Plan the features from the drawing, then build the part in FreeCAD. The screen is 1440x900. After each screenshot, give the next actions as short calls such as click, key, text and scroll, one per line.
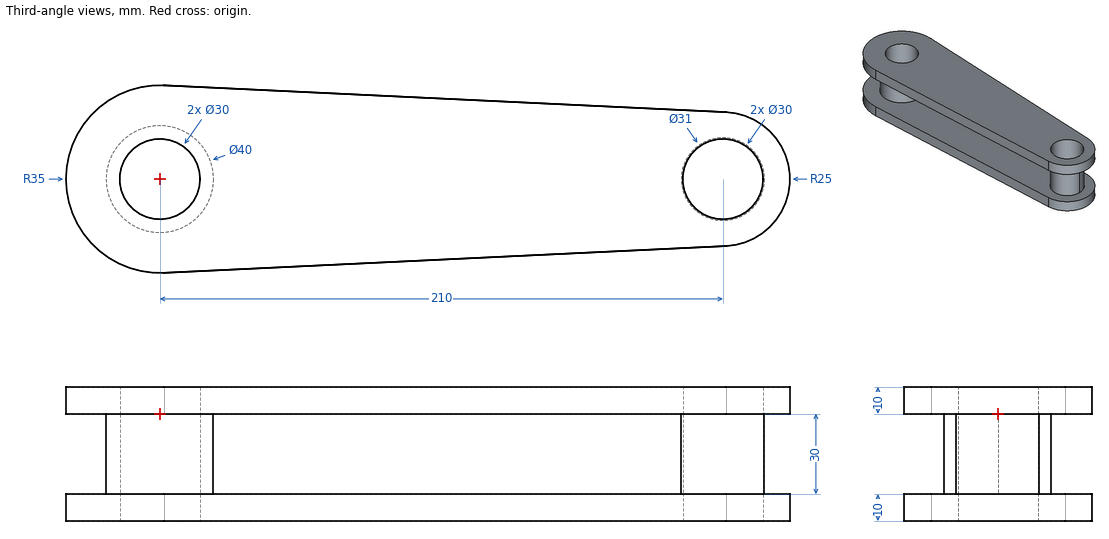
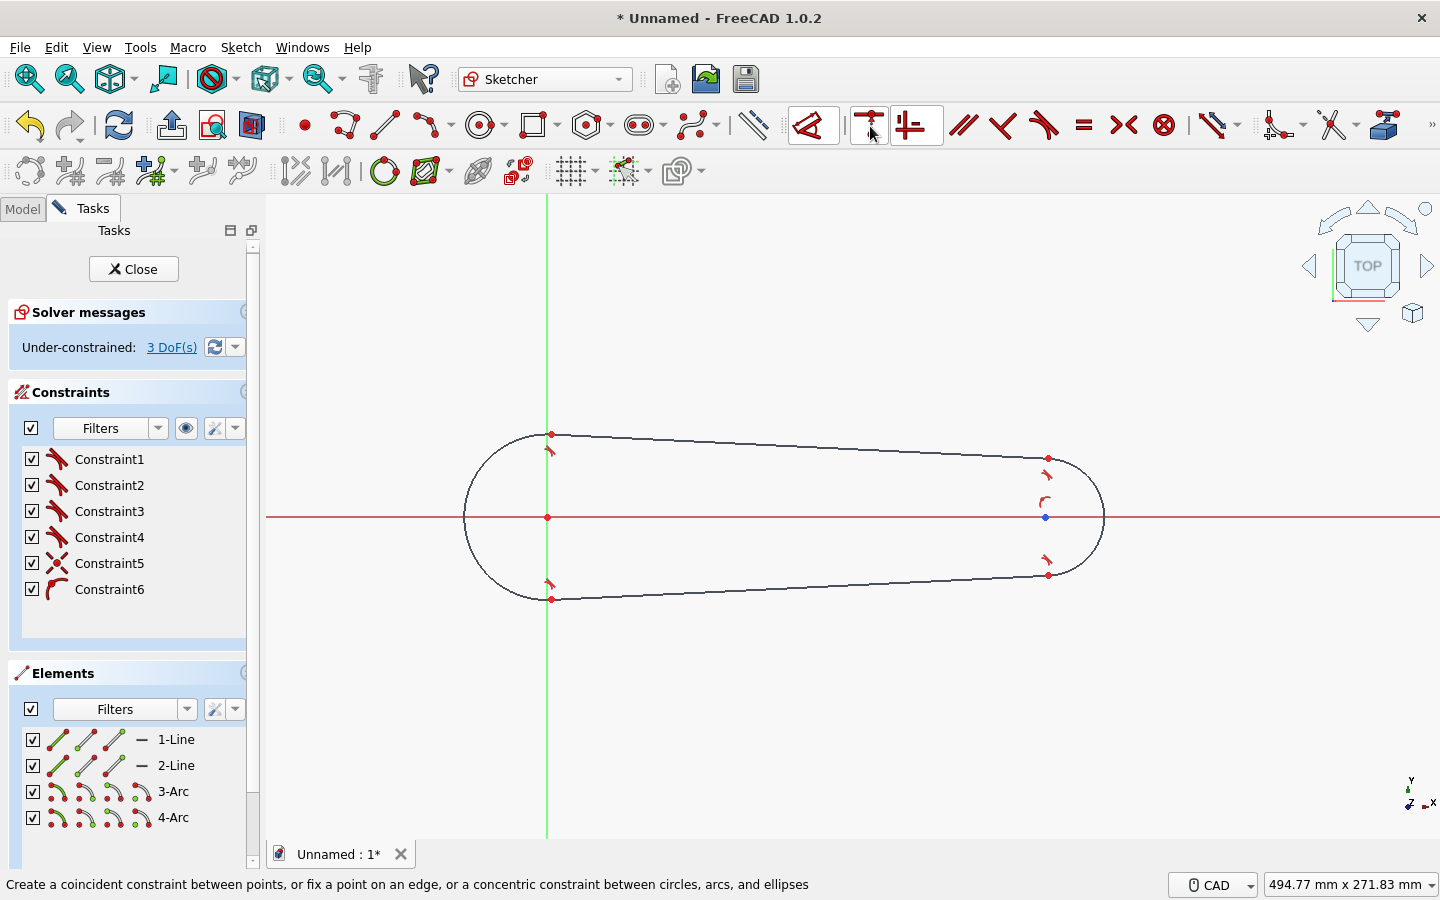
click(808, 126)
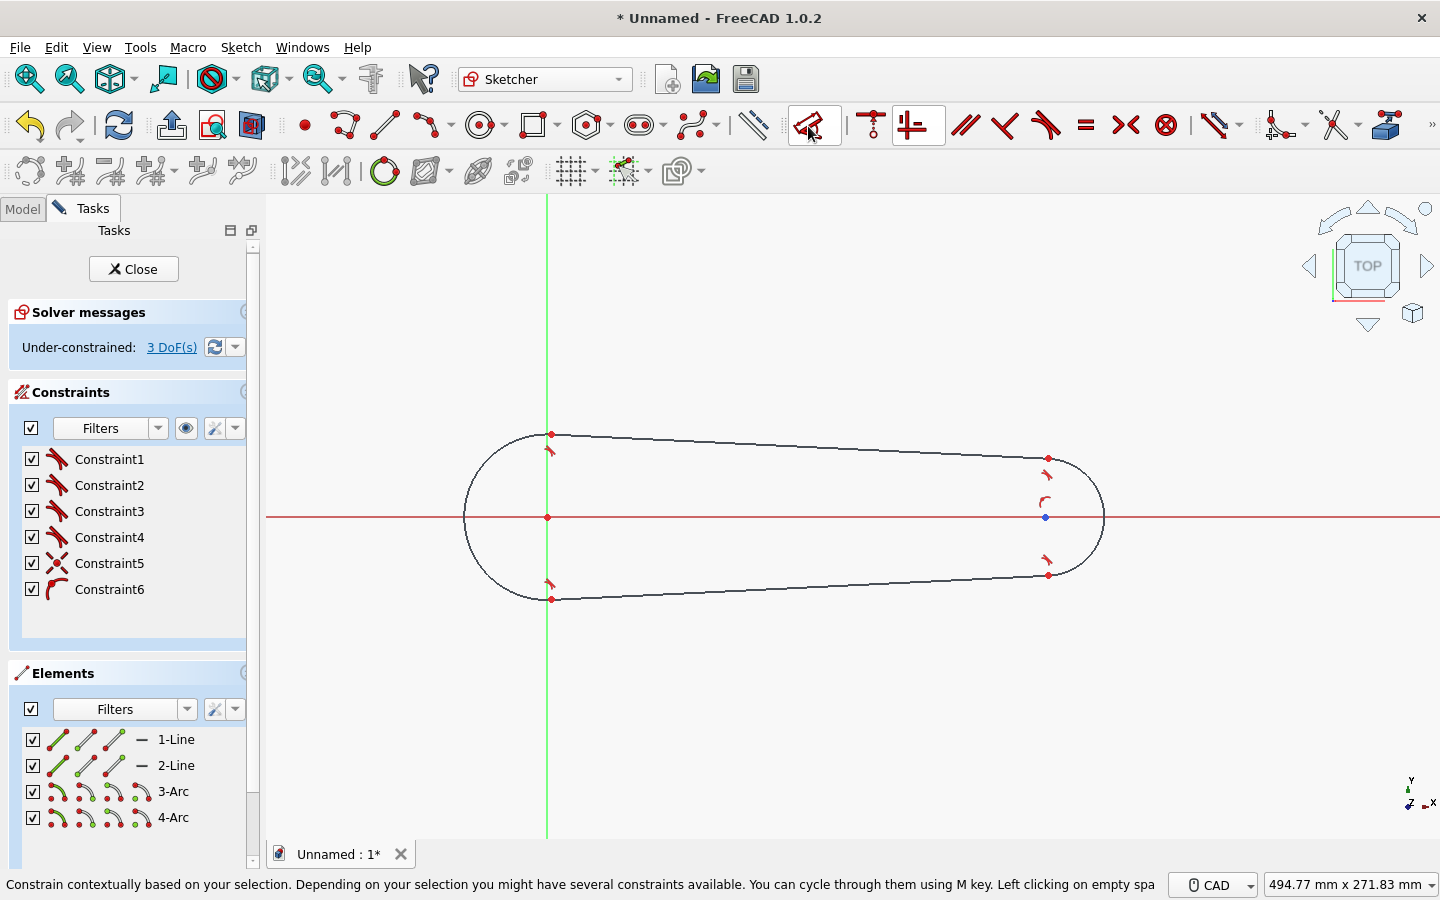
click(481, 467)
click(456, 448)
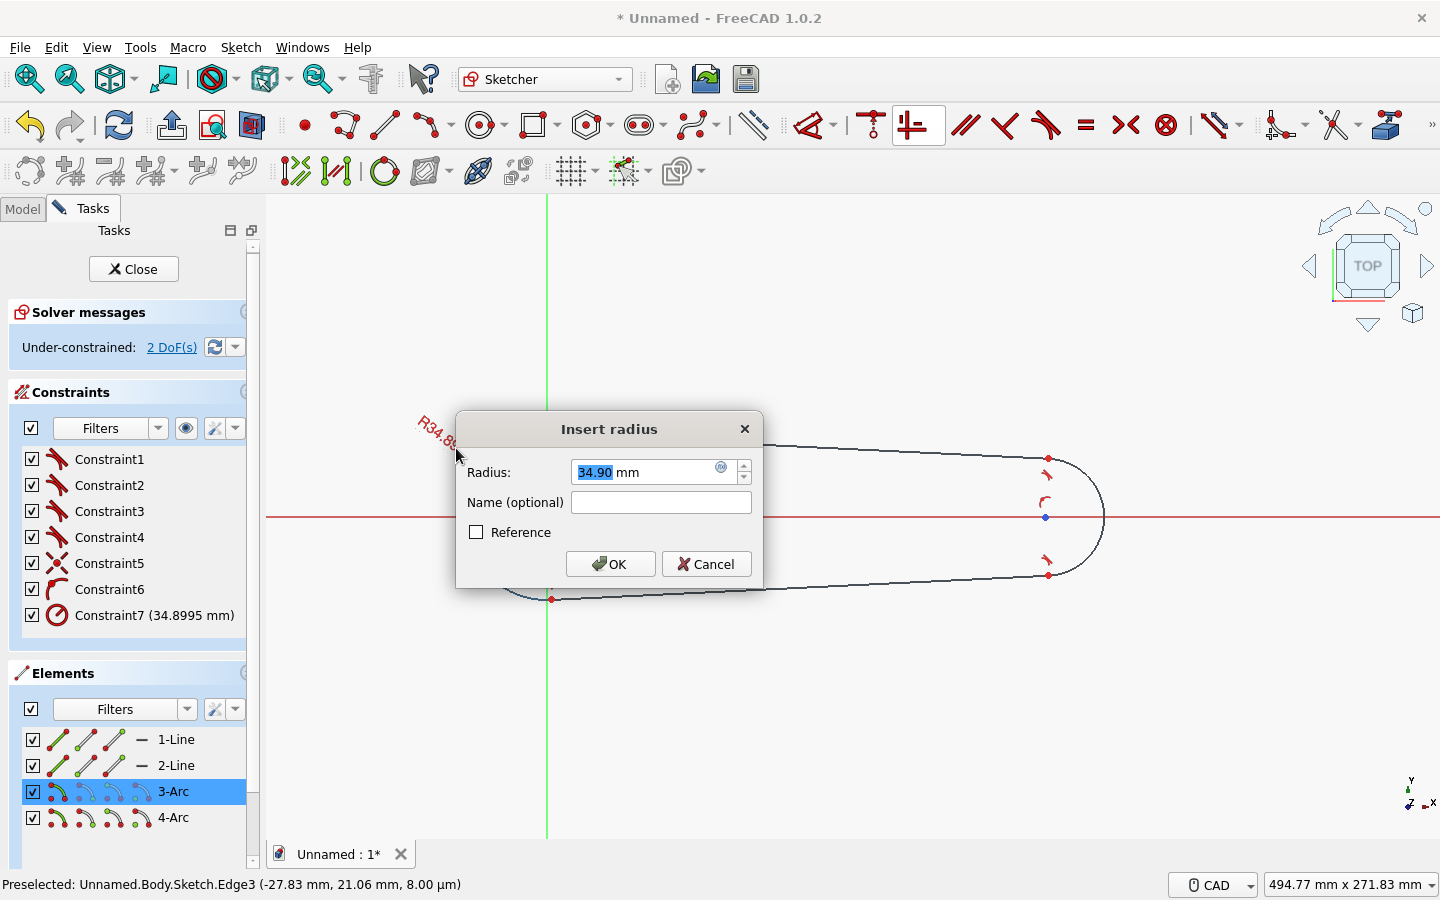
text(35)
key(Return)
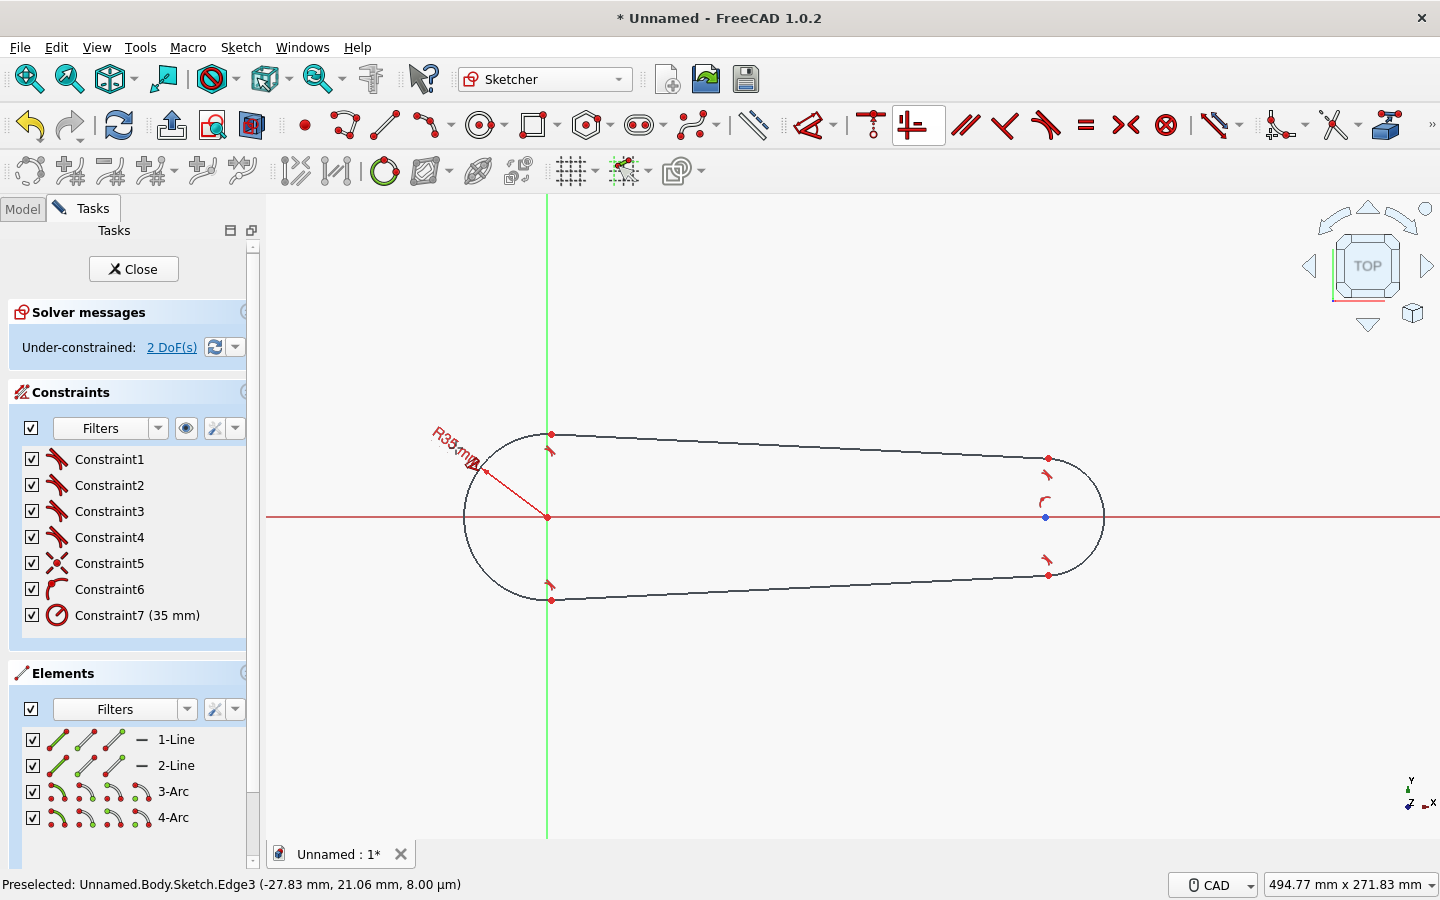
click(1094, 551)
click(1120, 569)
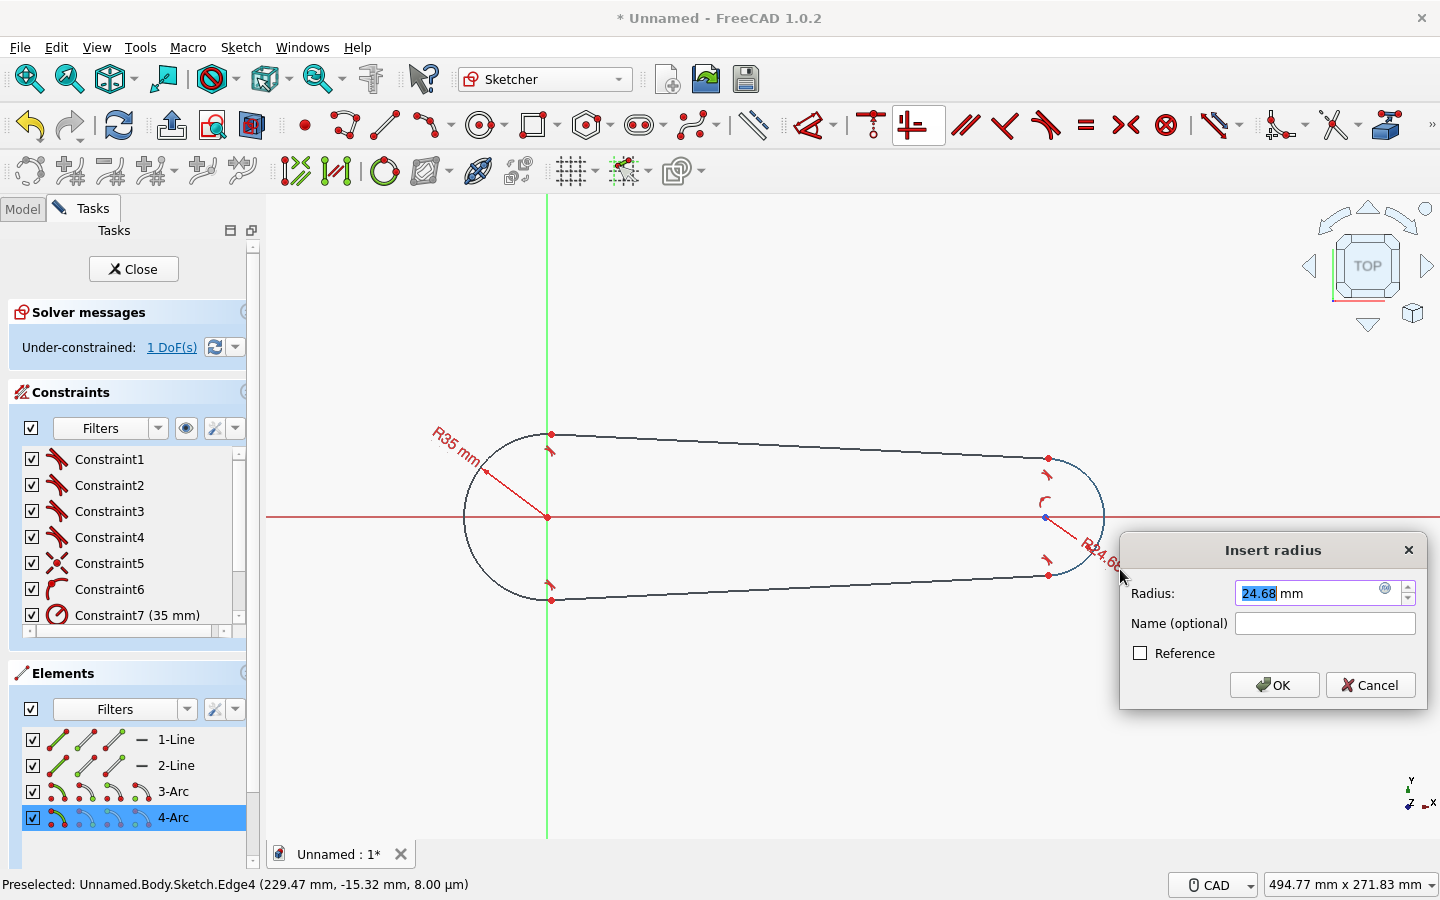
text(25)
key(Return)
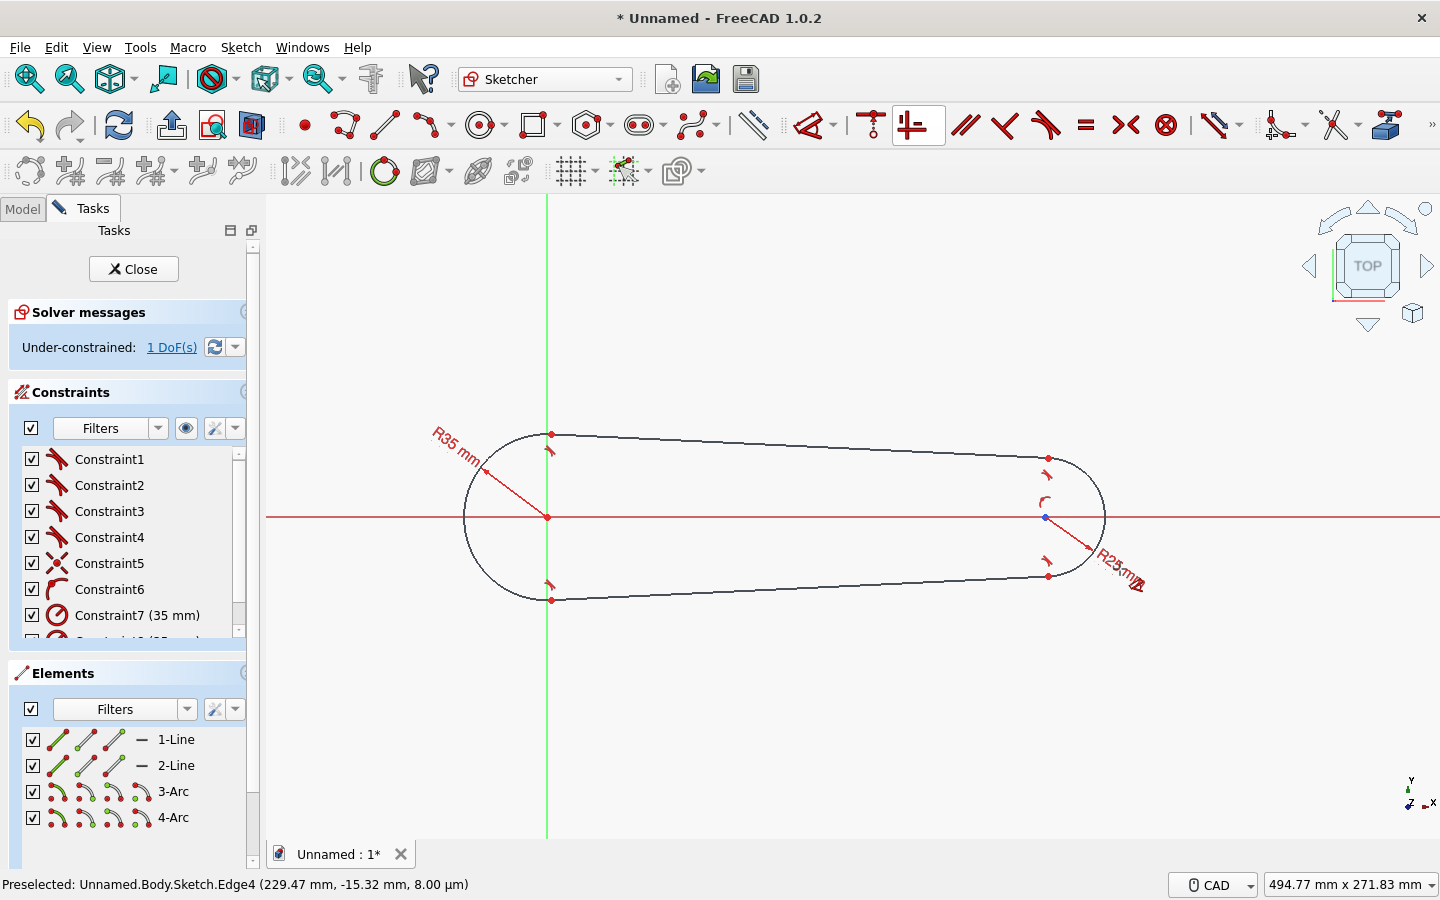
click(1046, 517)
click(796, 551)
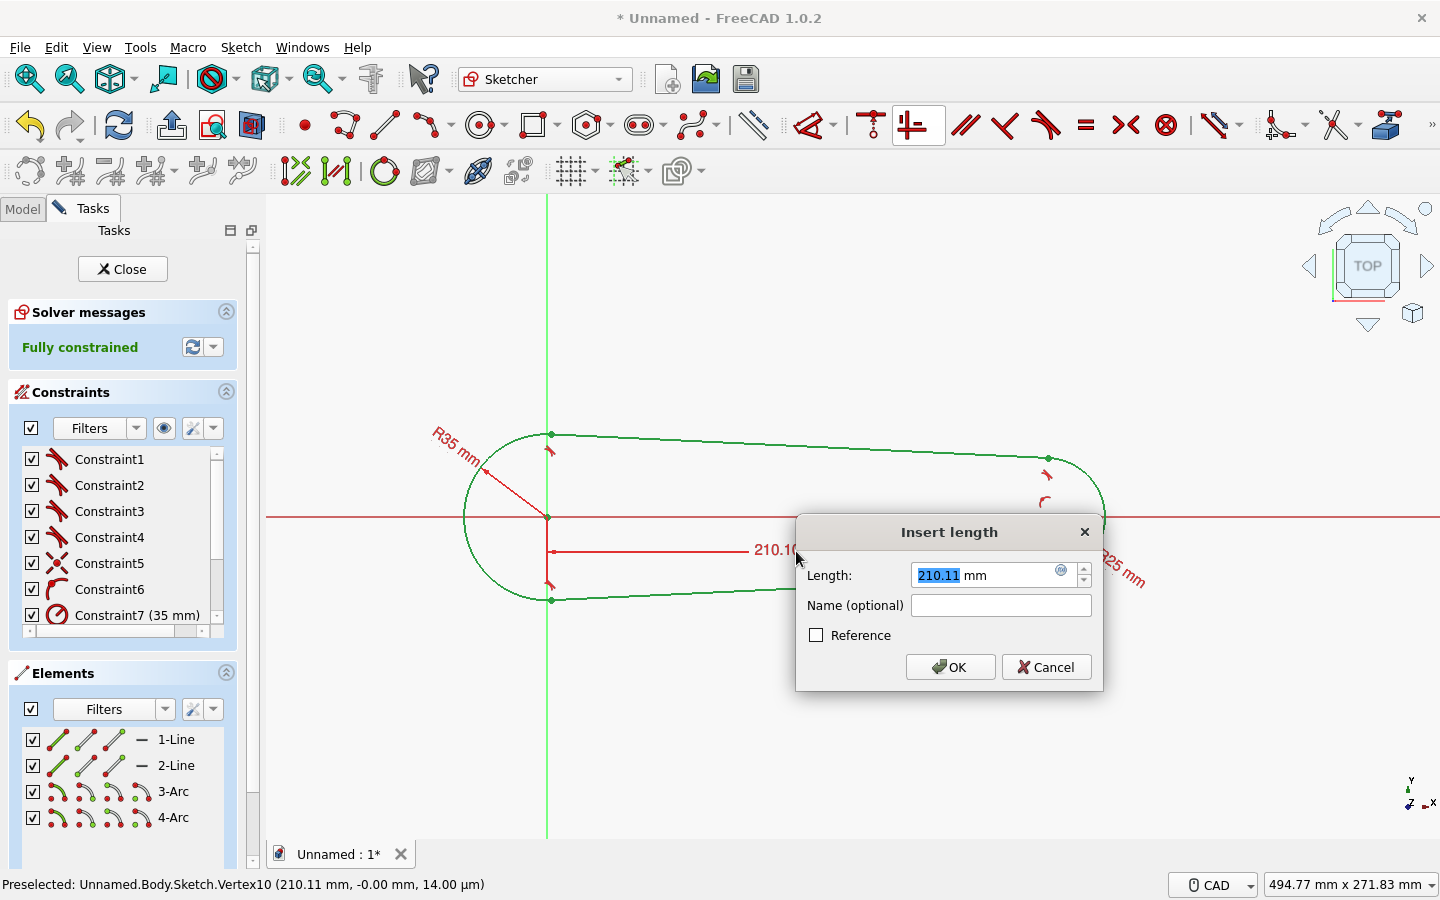
text(210)
key(Return)
key(Escape)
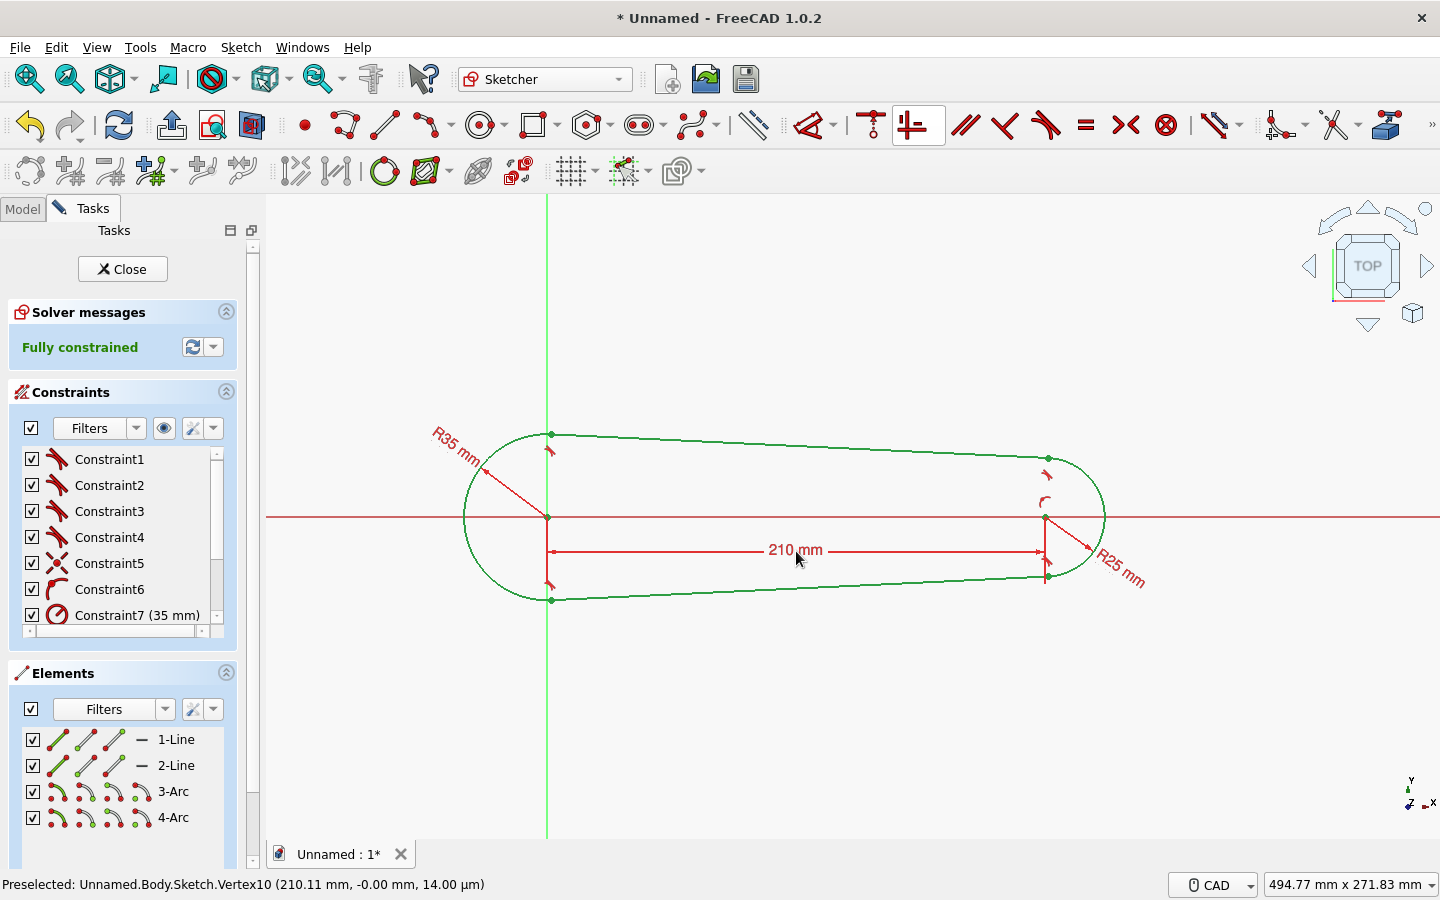
click(123, 269)